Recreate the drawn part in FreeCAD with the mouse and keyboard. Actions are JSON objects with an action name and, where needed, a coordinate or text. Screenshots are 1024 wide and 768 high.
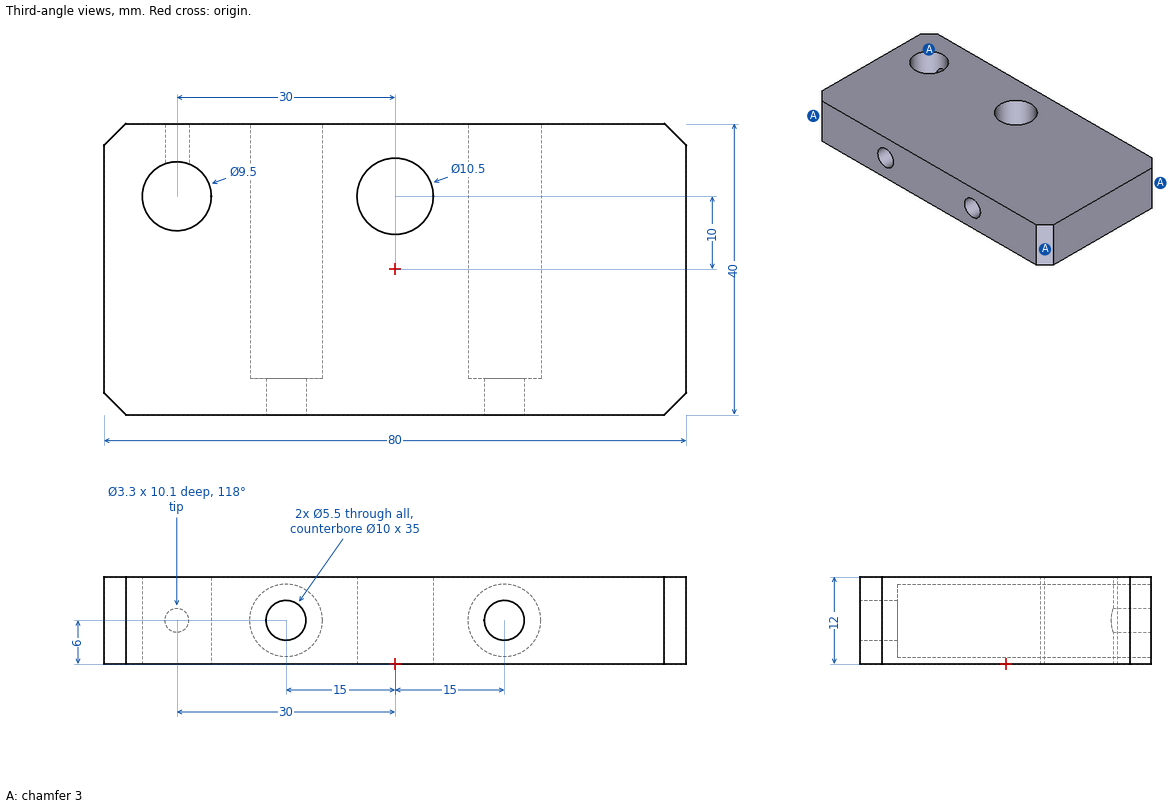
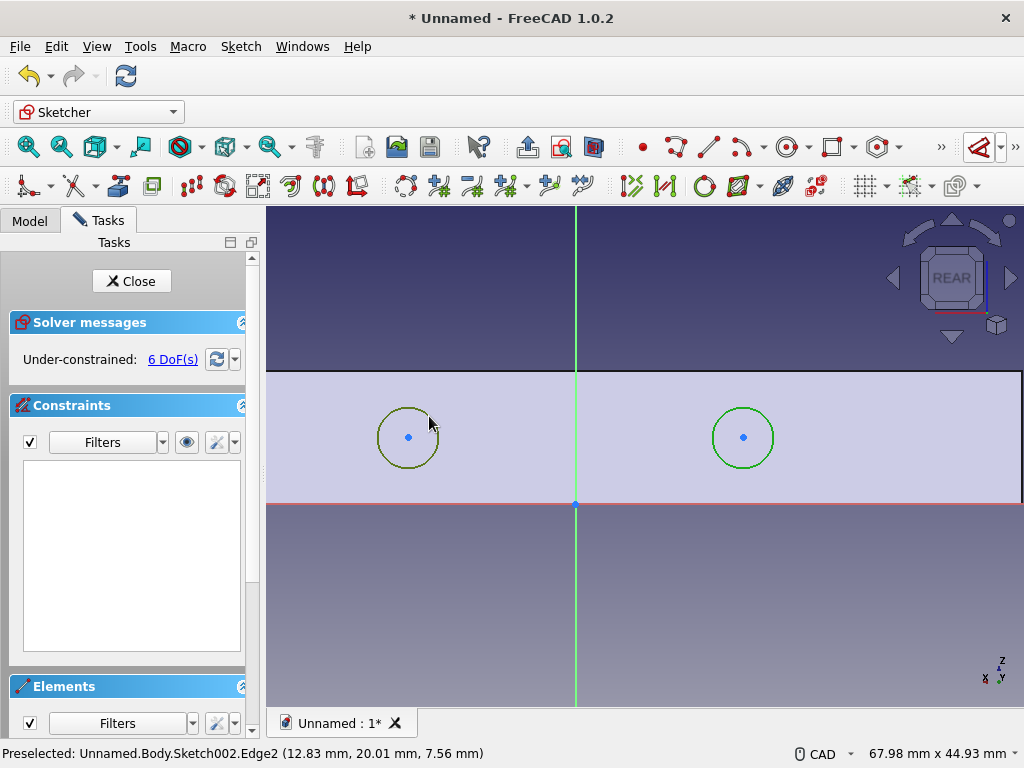
{"action": "key", "text": "e"}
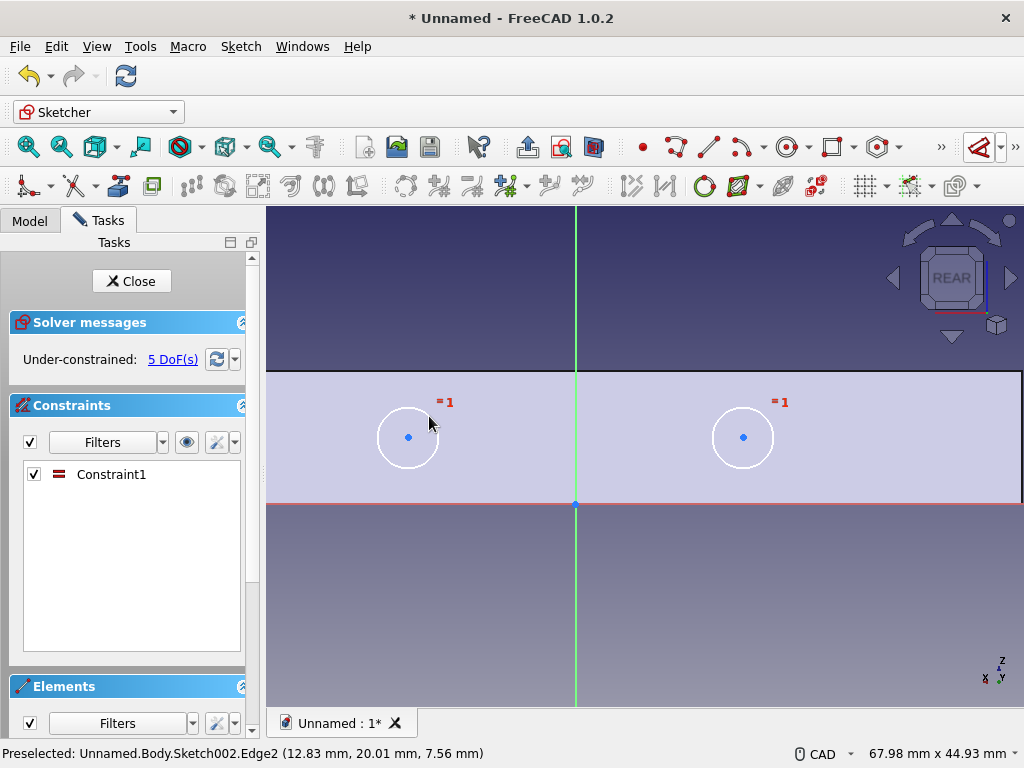
{"action": "left_click", "coordinate": [743, 438]}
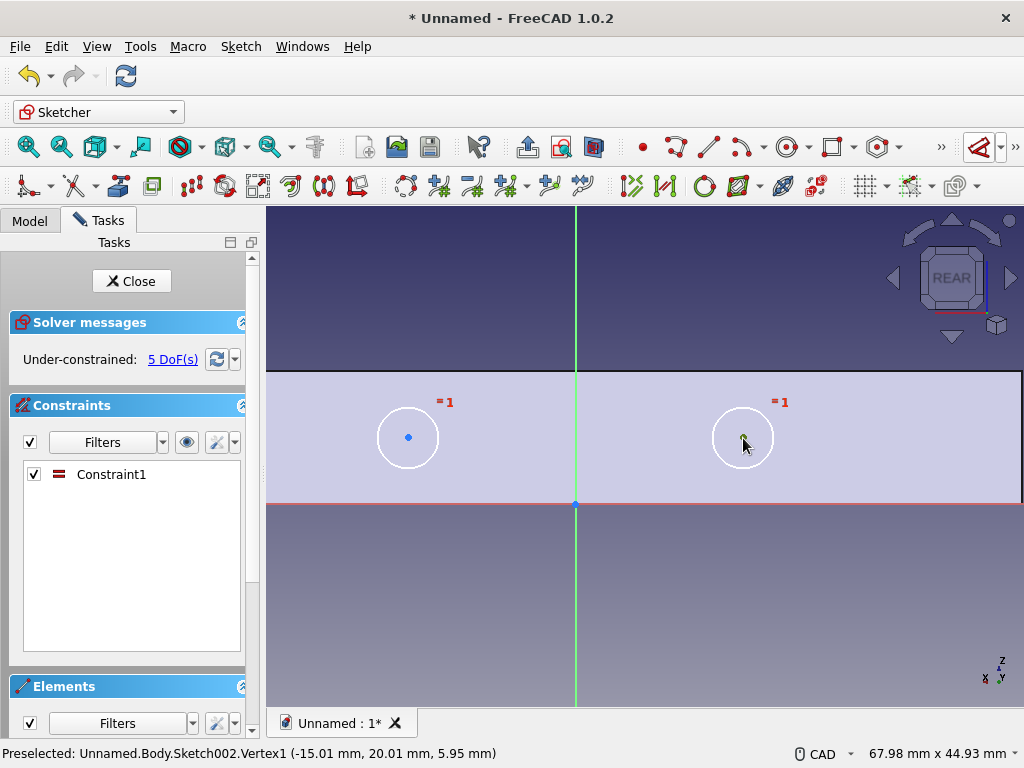
{"action": "left_click", "coordinate": [408, 438]}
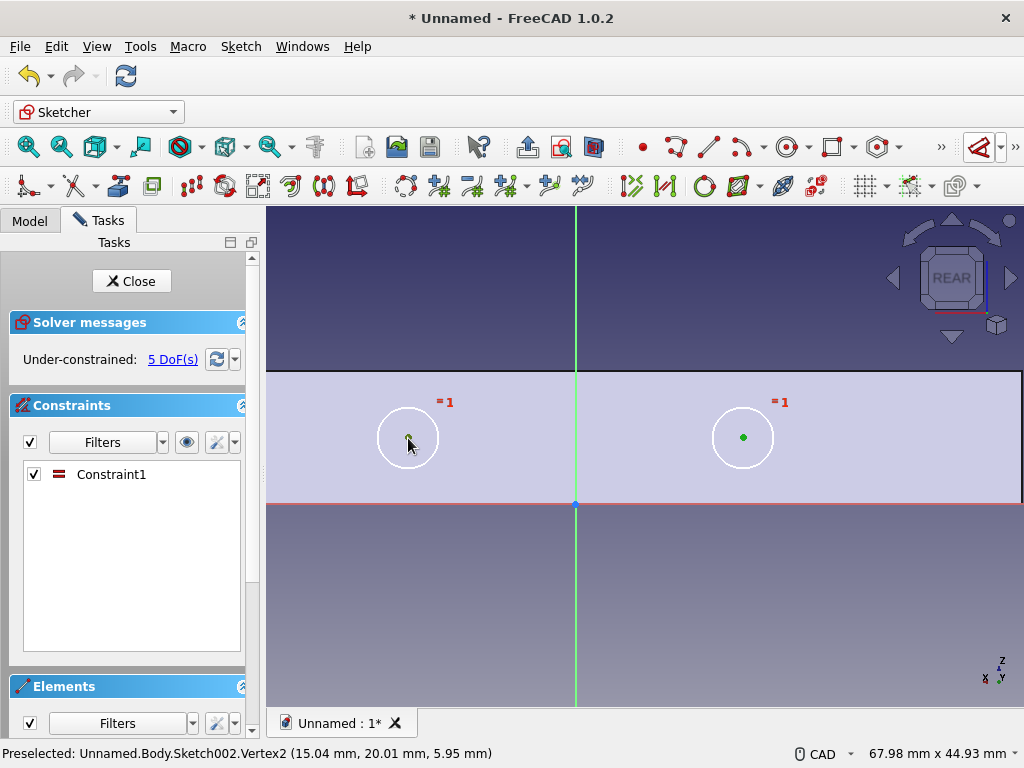
{"action": "key", "text": "h"}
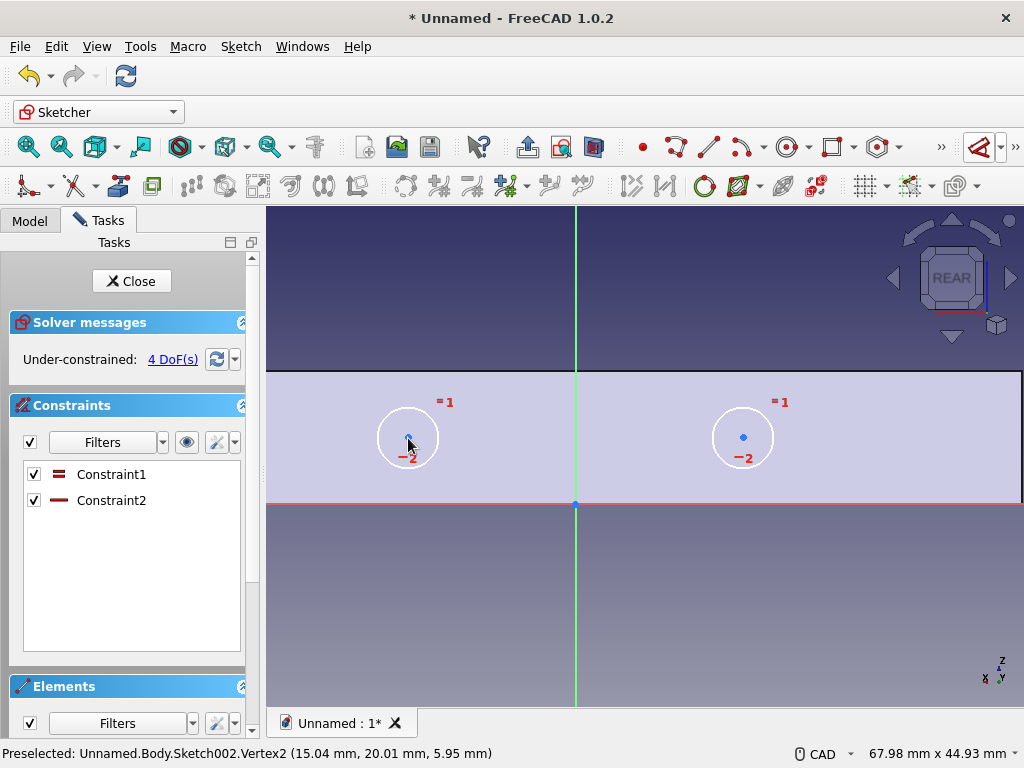
{"action": "left_click", "coordinate": [764, 416]}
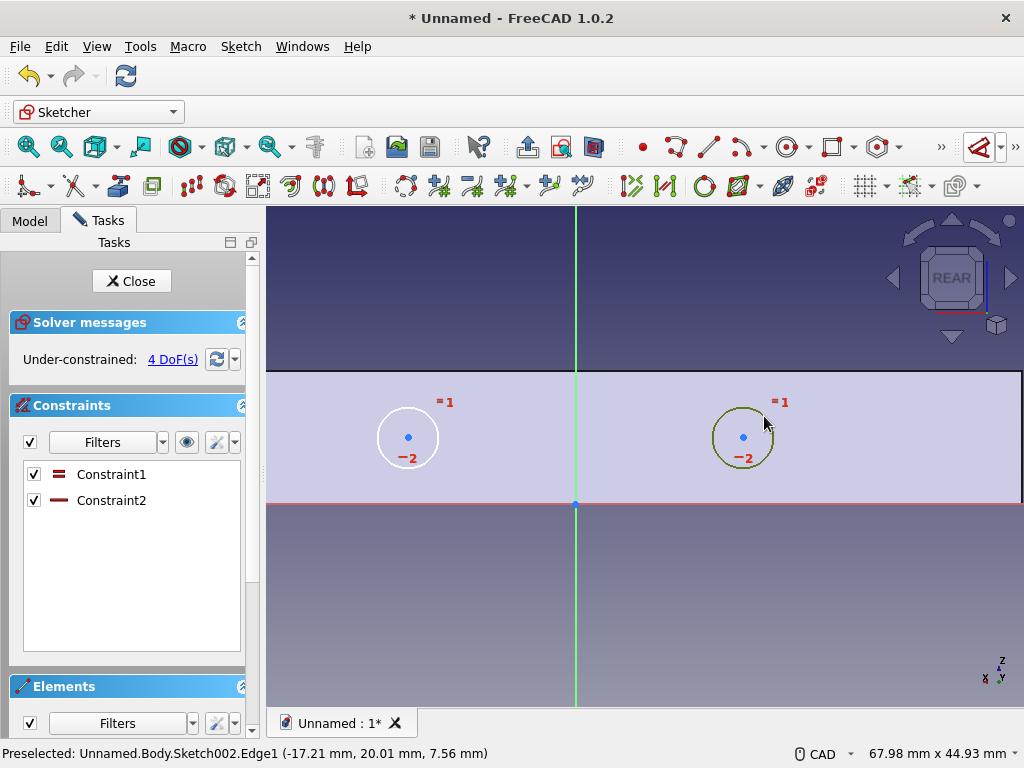
{"action": "key", "text": "k o"}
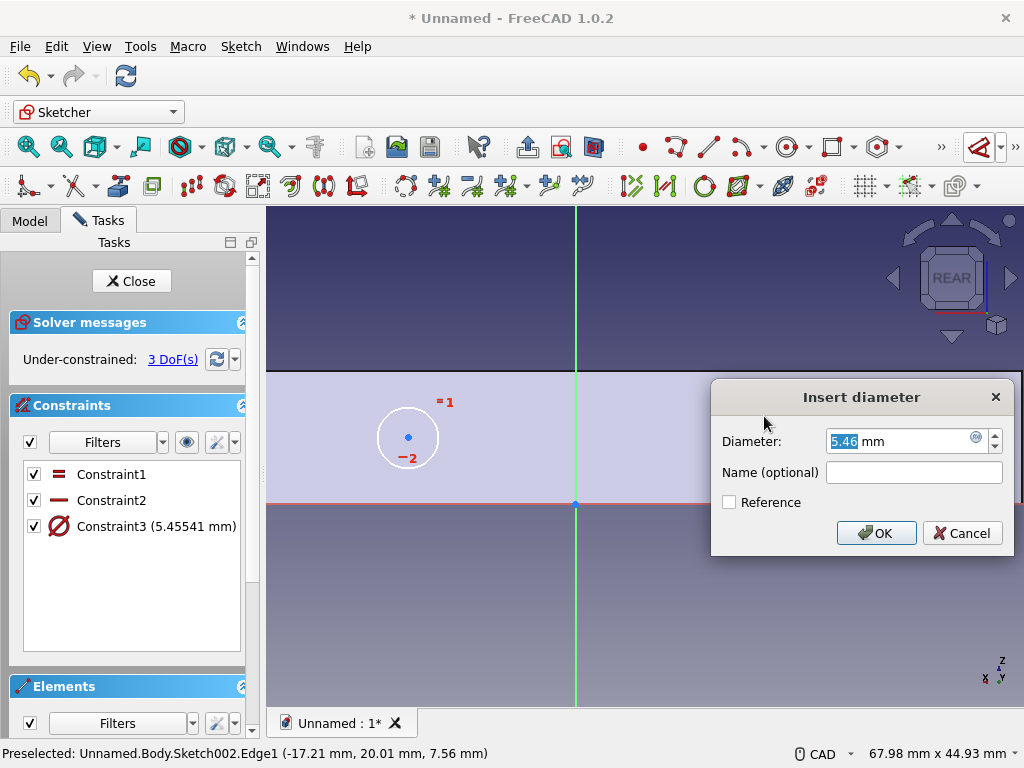
{"action": "type", "text": "5.5"}
{"action": "key", "text": "Return"}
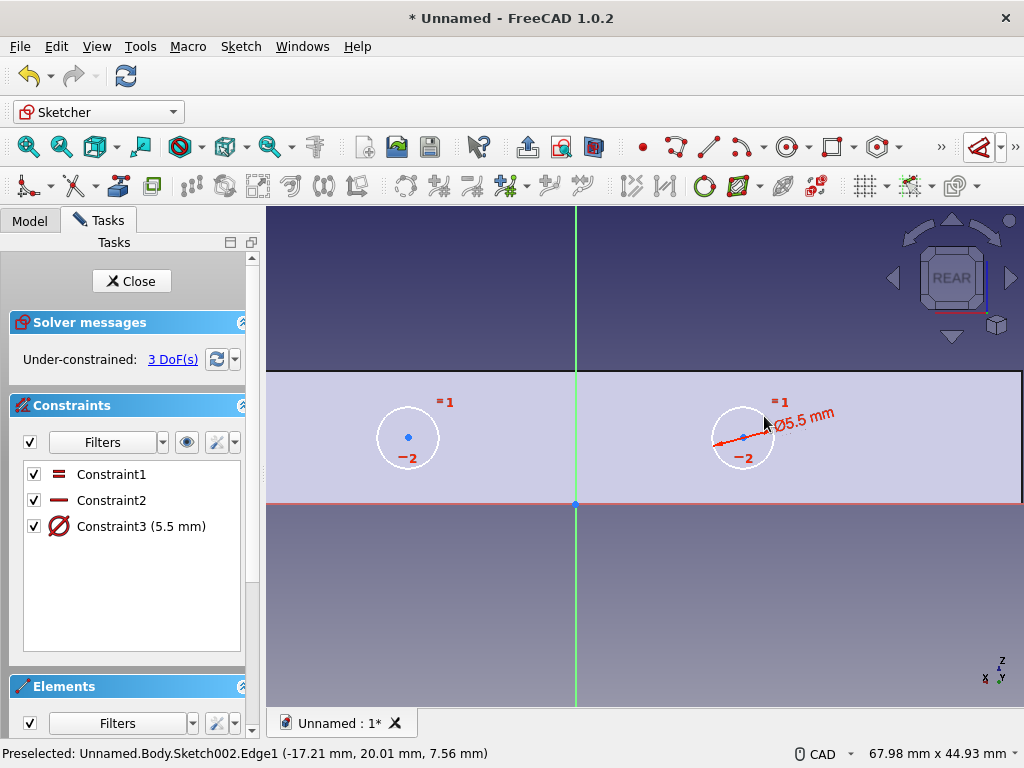
{"action": "left_click", "coordinate": [743, 438]}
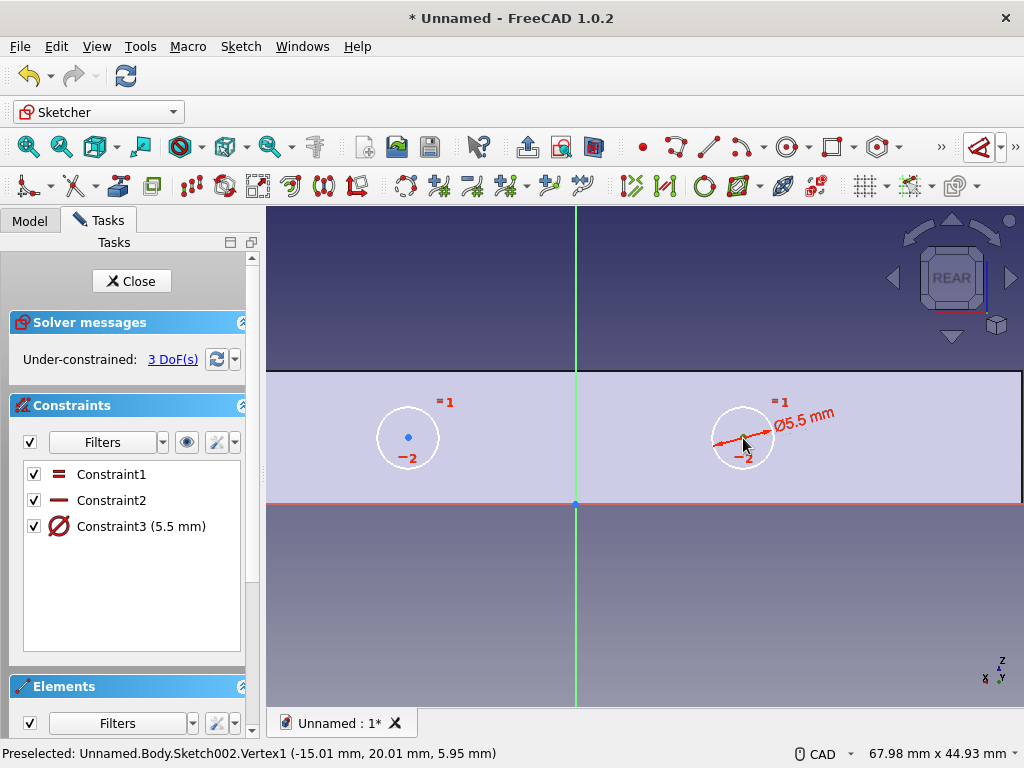
{"action": "left_click", "coordinate": [1000, 148]}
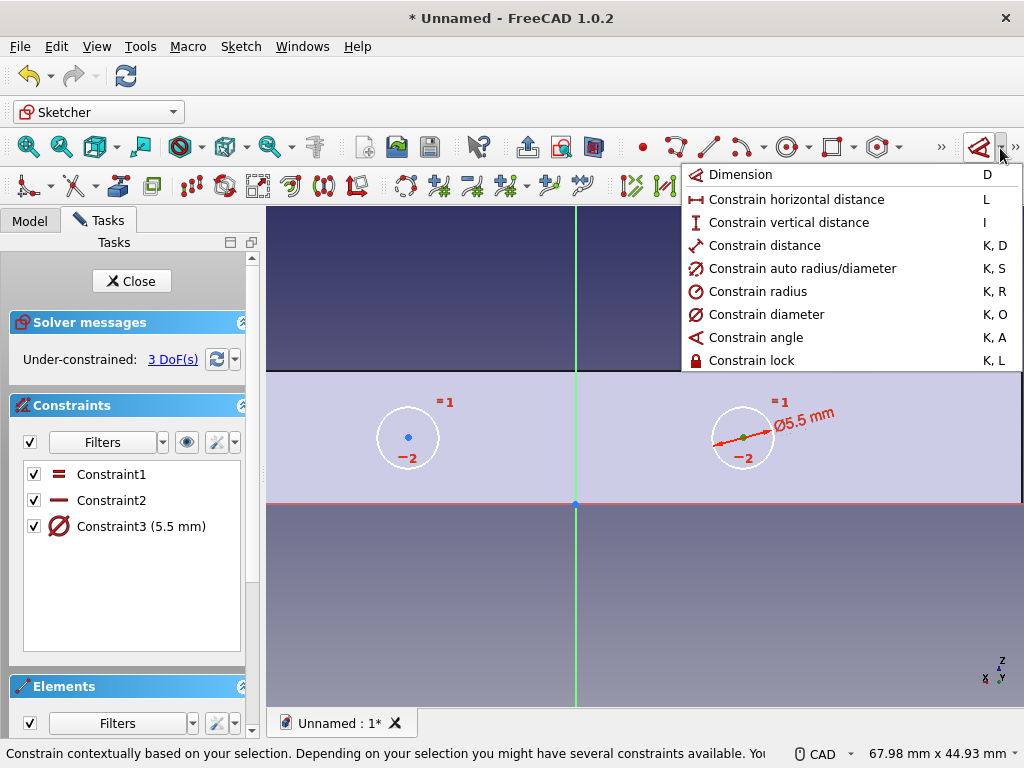
{"action": "left_click", "coordinate": [852, 222]}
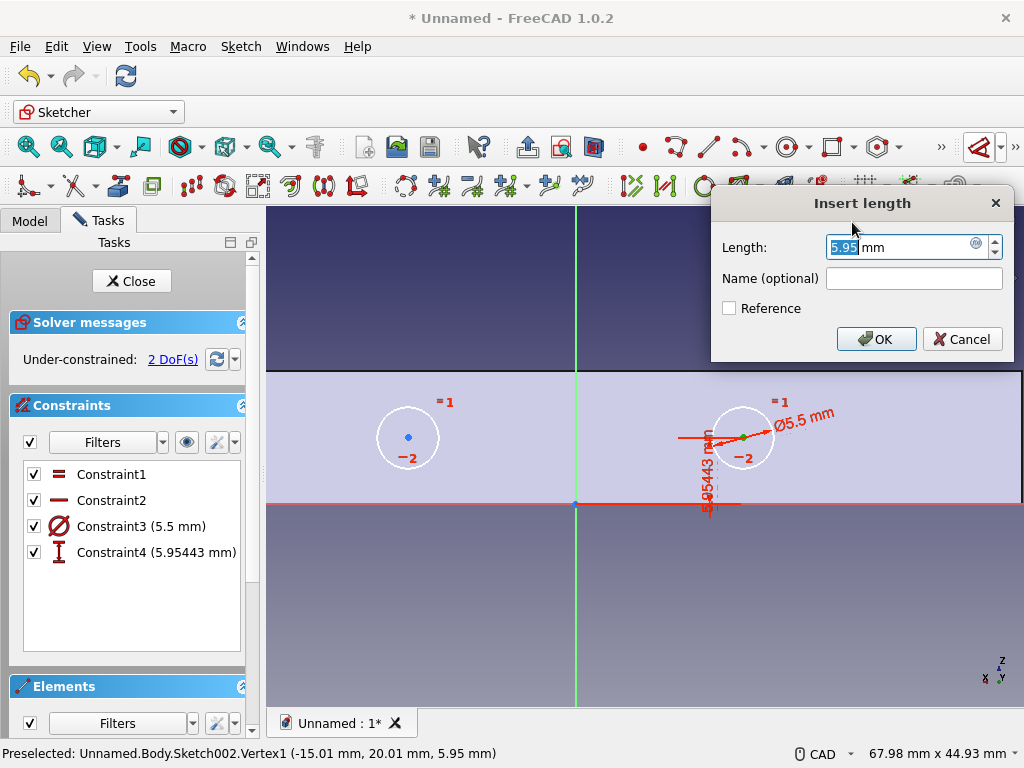
{"action": "type", "text": "6"}
{"action": "key", "text": "Return"}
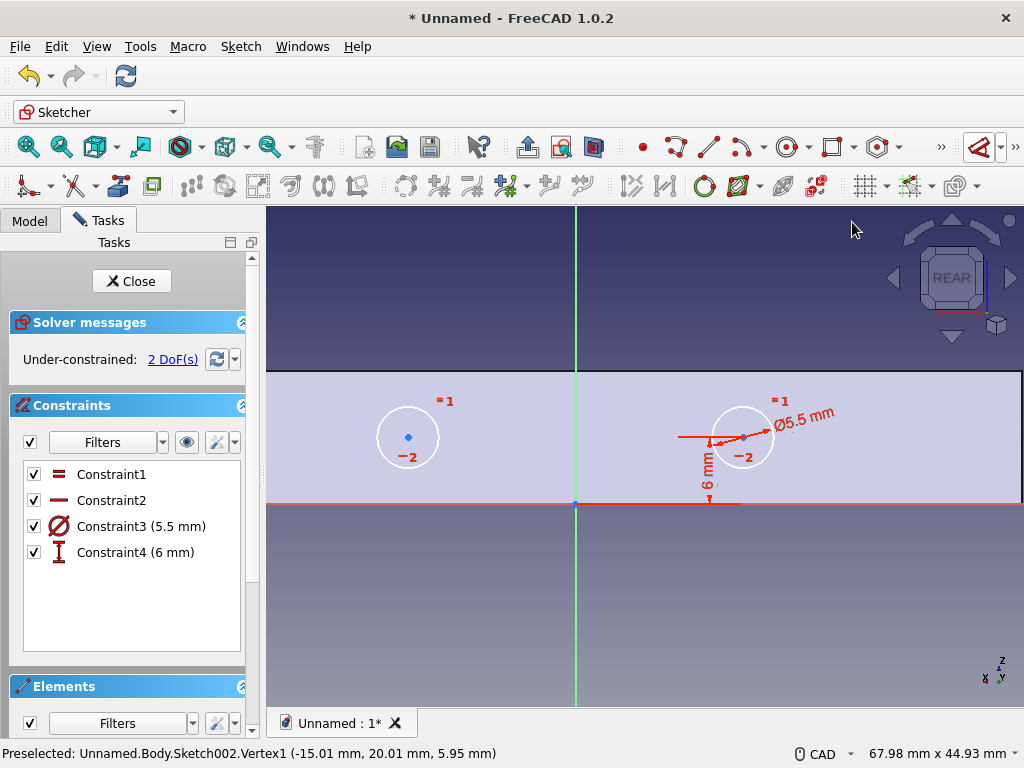
{"action": "left_click", "coordinate": [743, 437]}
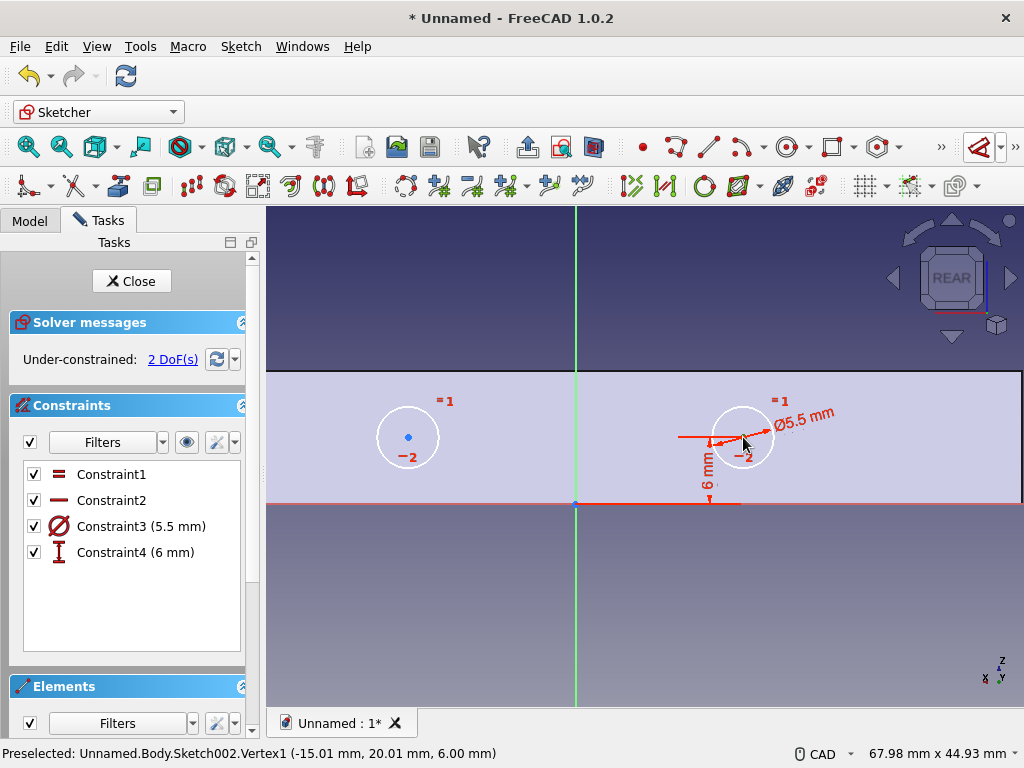
{"action": "left_click", "coordinate": [1000, 148]}